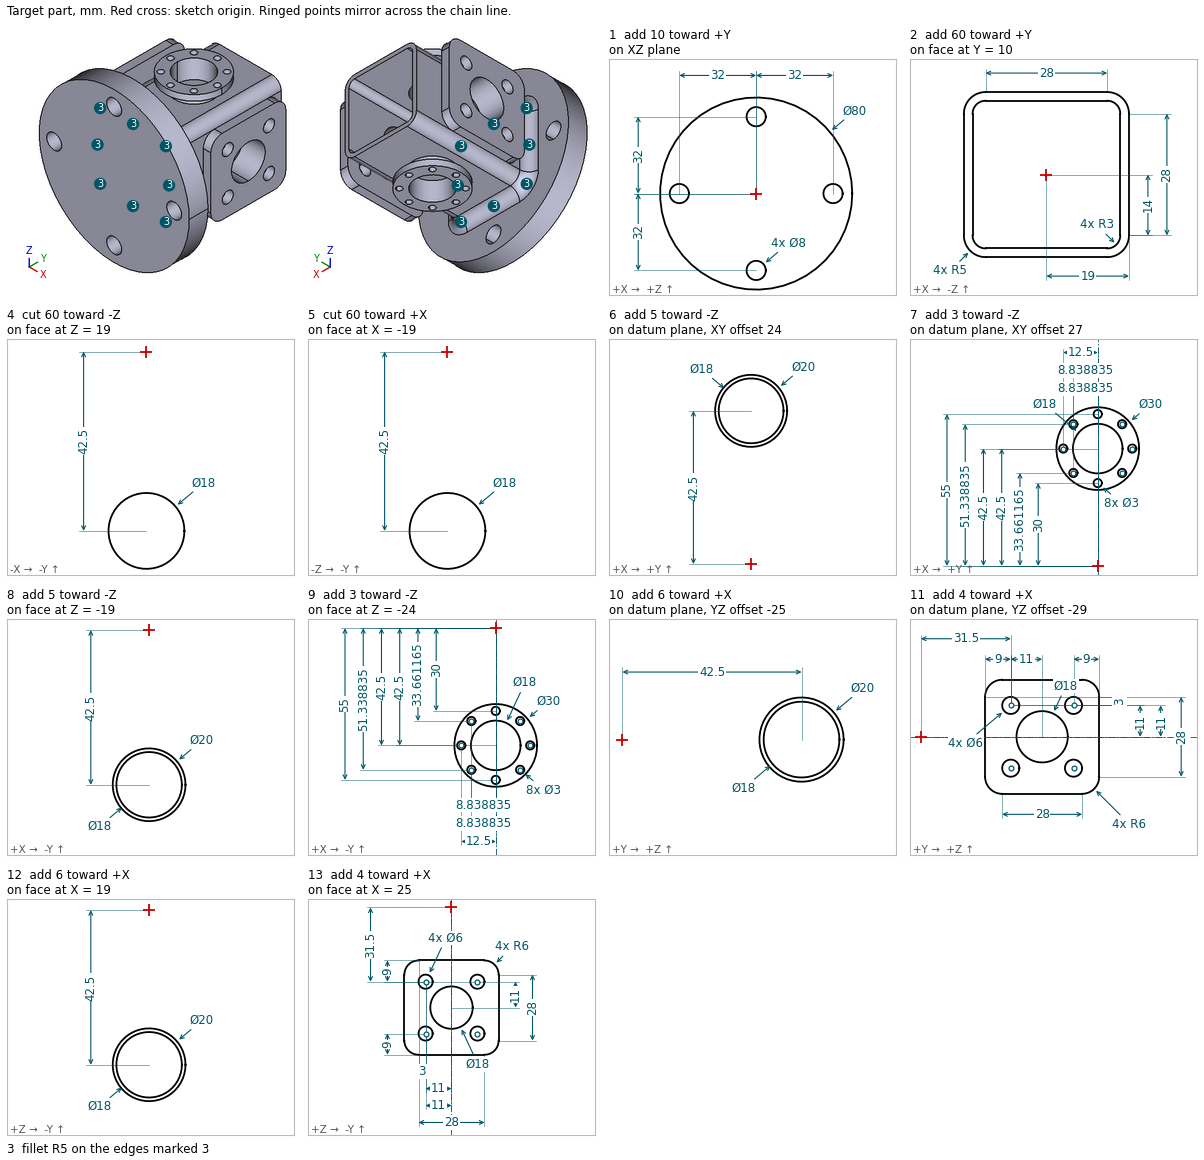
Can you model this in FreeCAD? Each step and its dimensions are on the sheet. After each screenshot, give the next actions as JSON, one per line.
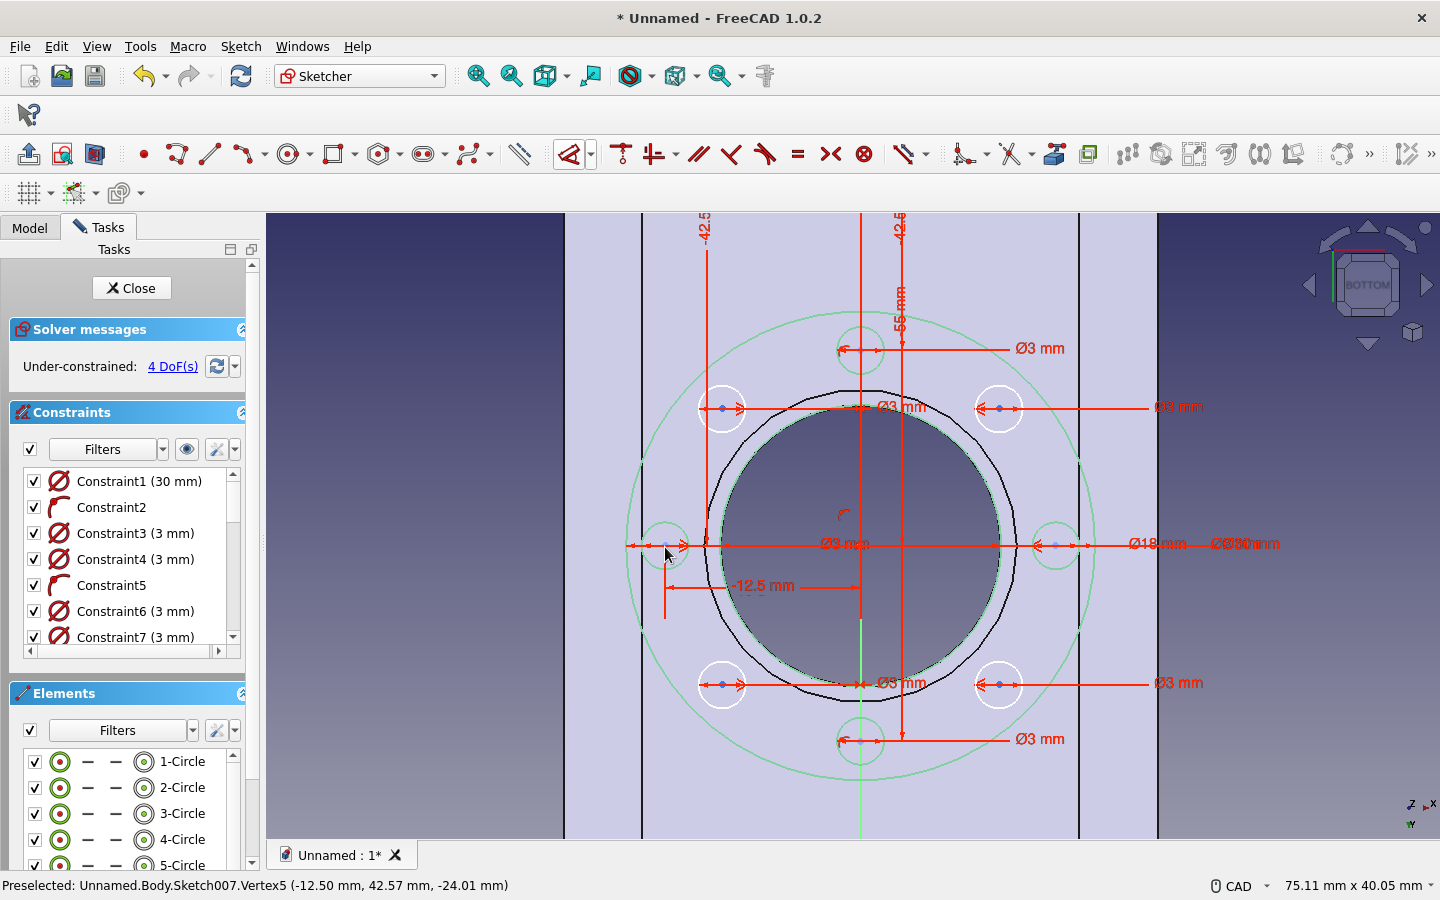
{"action": "left_click", "coordinate": [722, 685]}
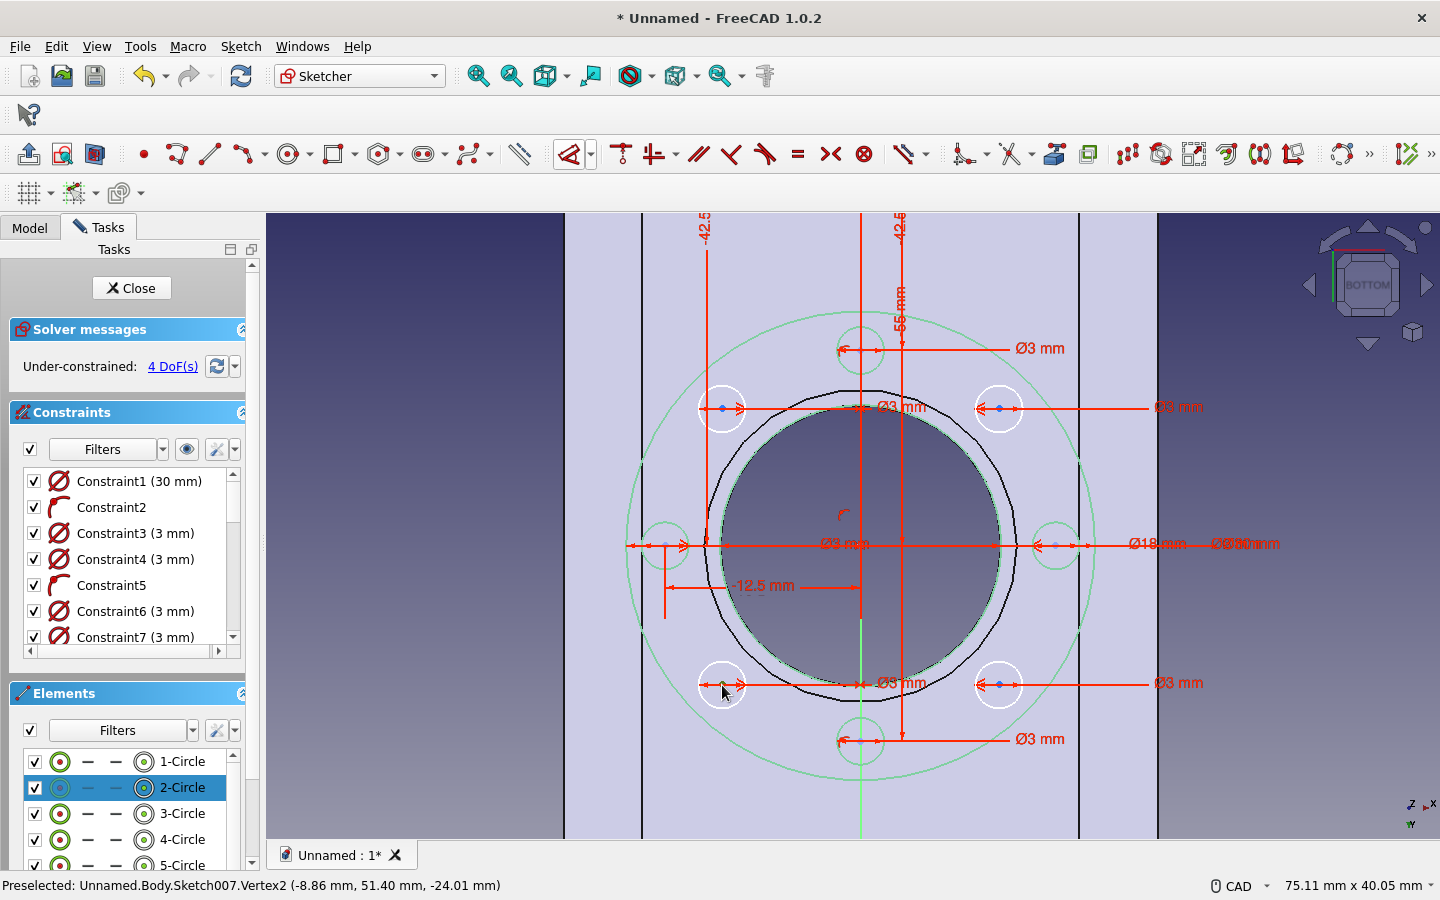
{"action": "key", "text": "l"}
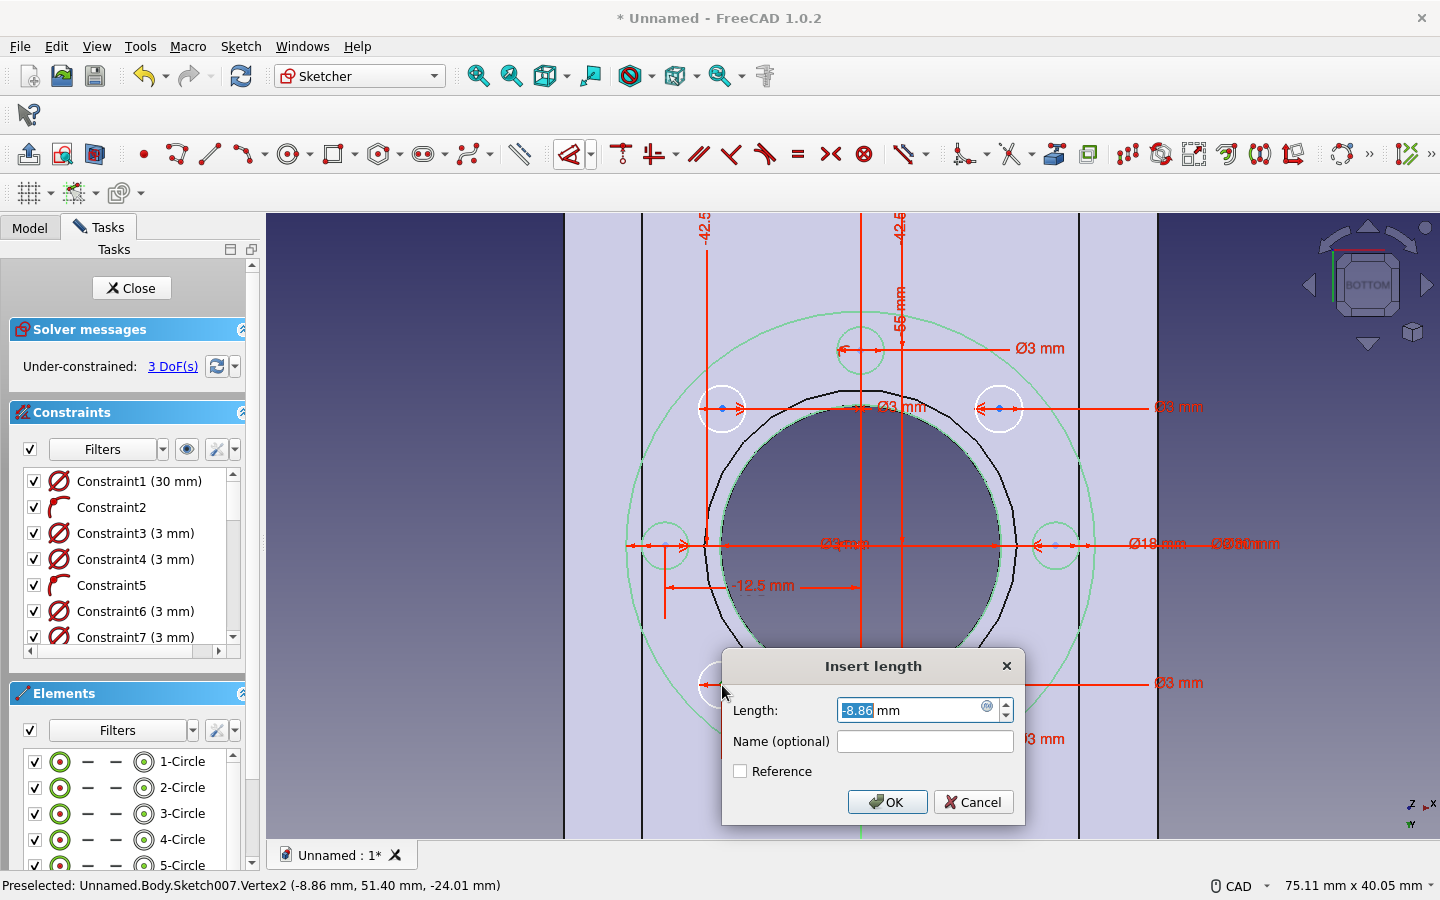
{"action": "type", "text": "-8.838835"}
{"action": "key", "text": "Return"}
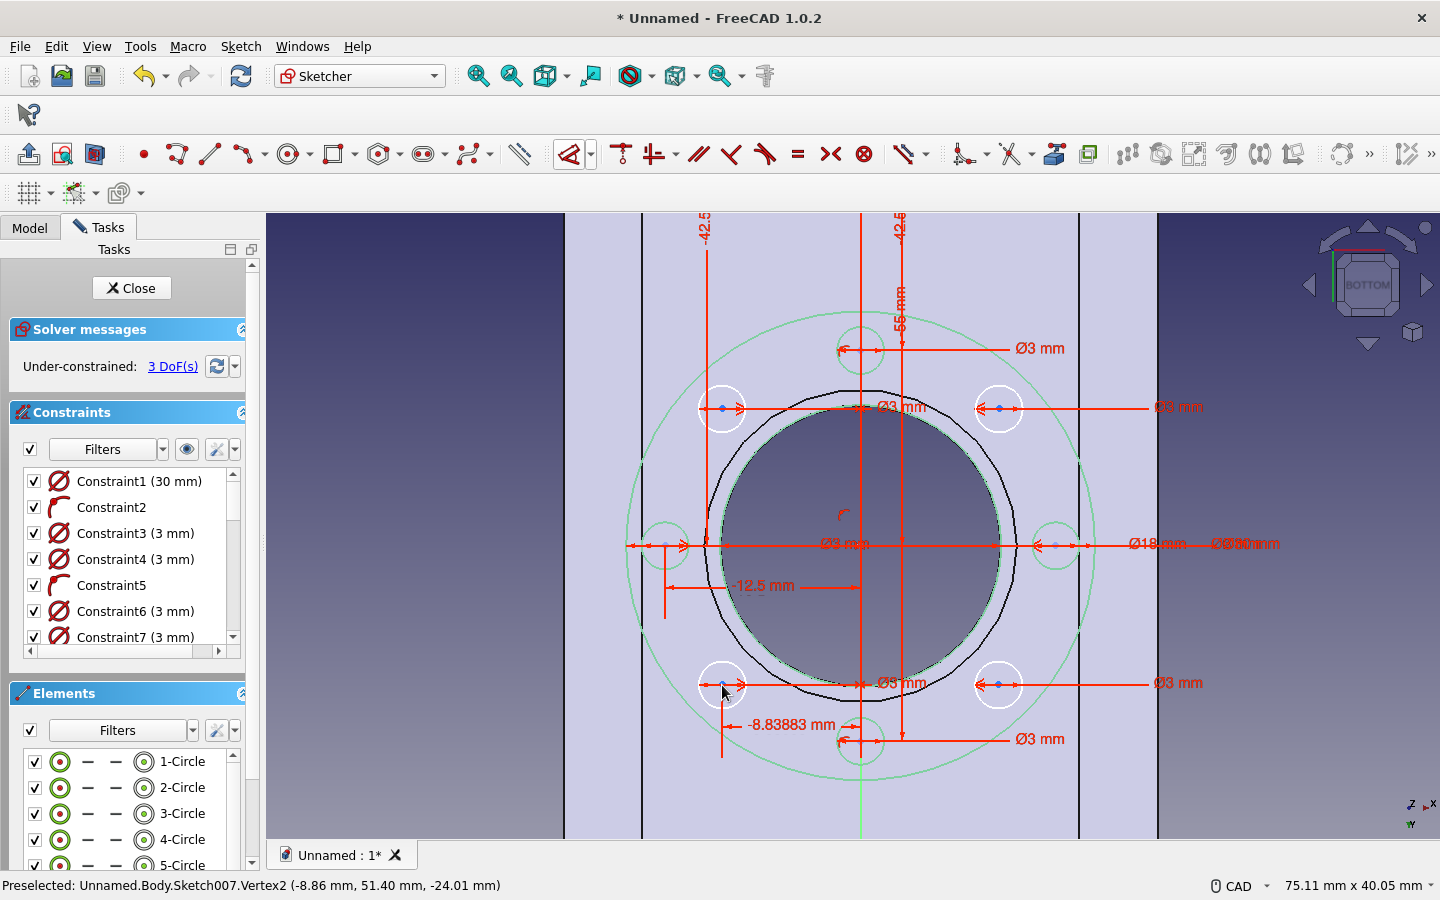
{"action": "left_click", "coordinate": [722, 409]}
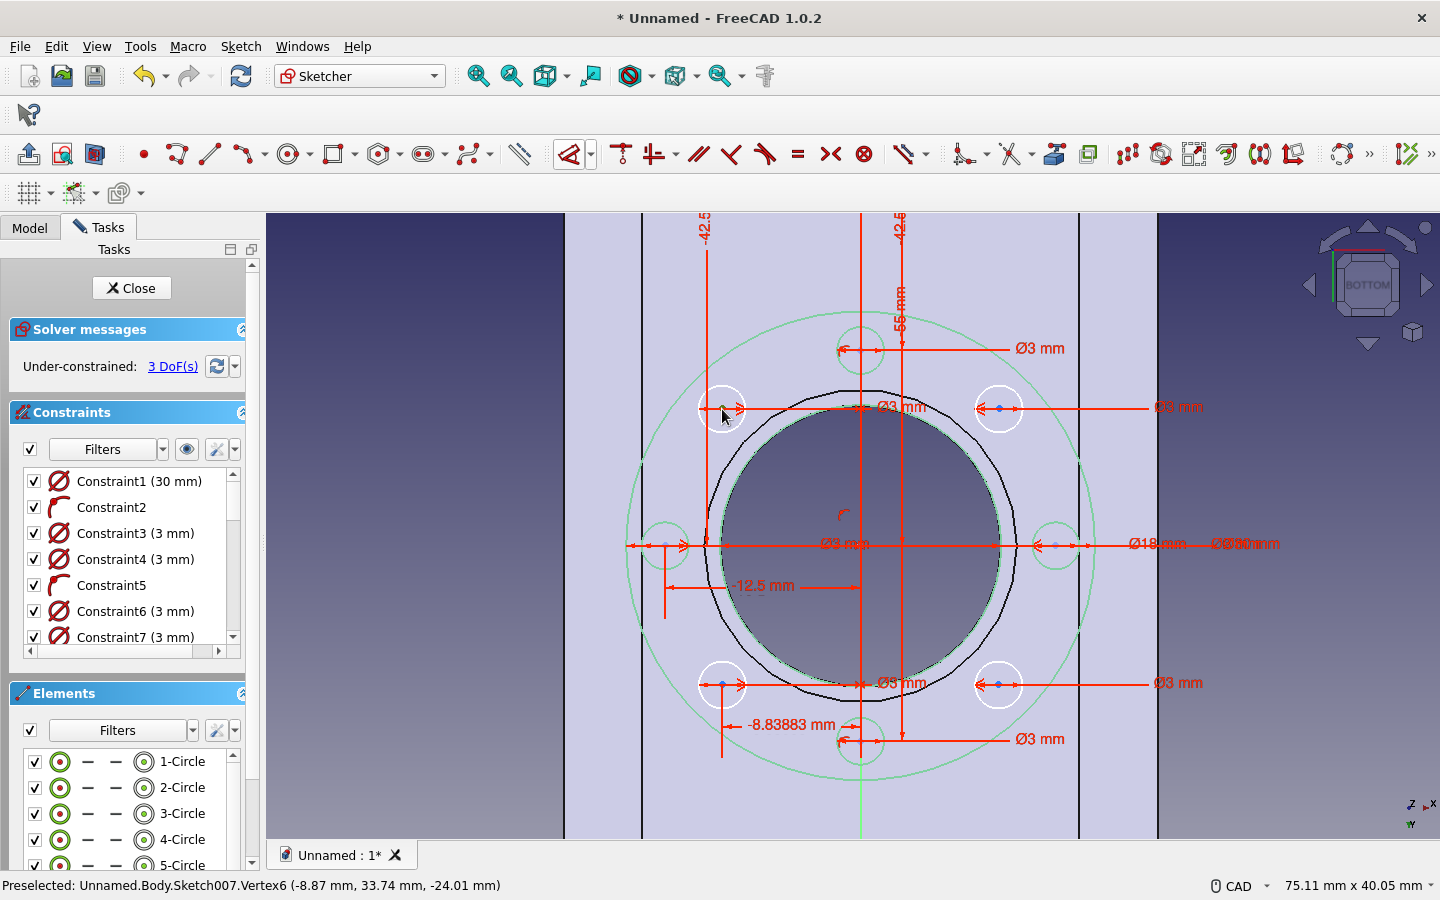
{"action": "key", "text": "l"}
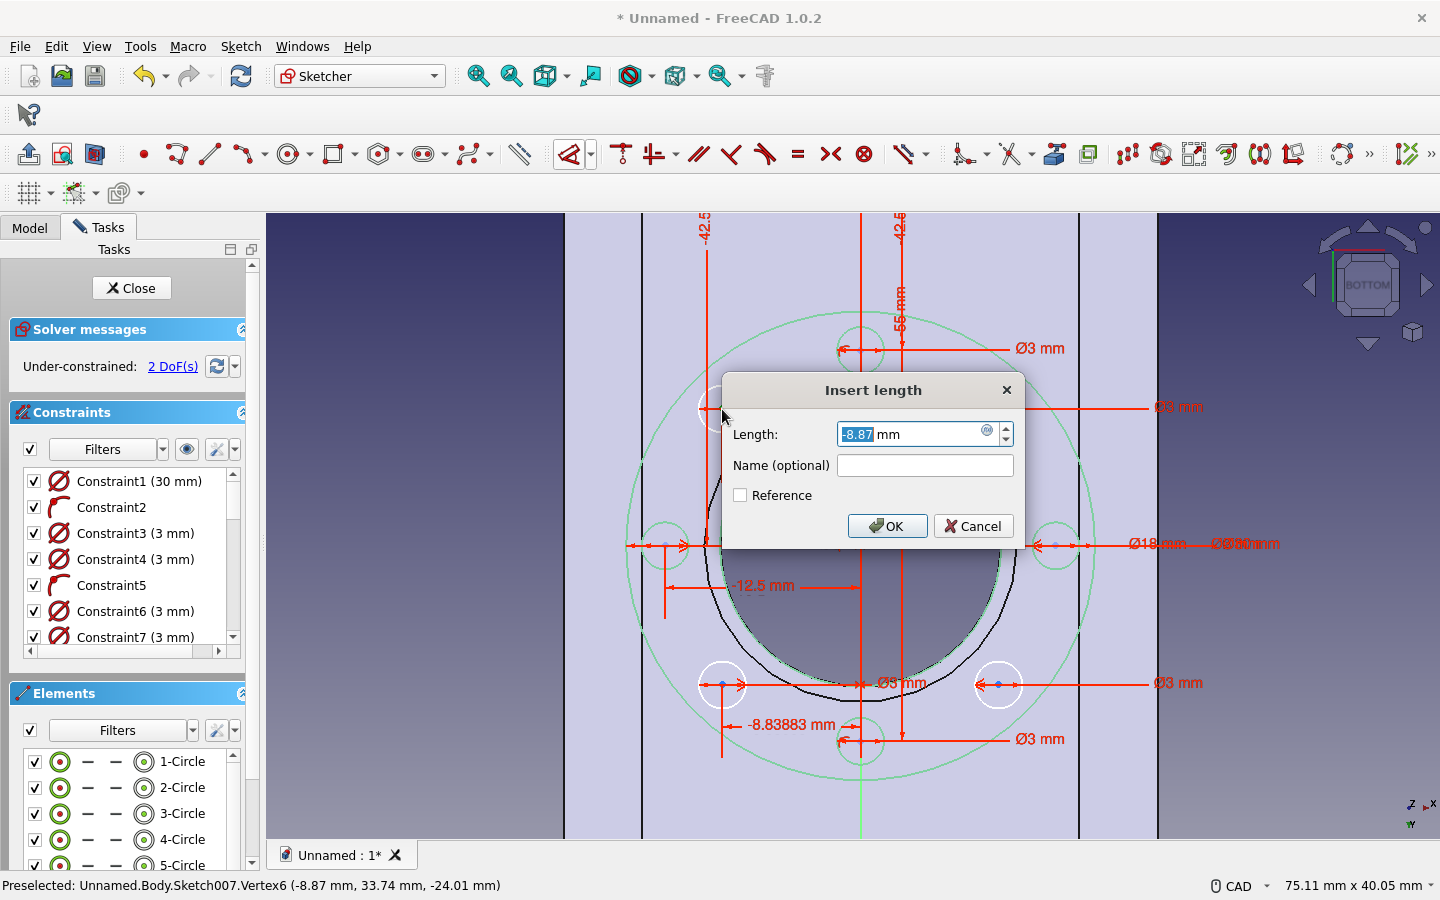
{"action": "type", "text": "-8.838835"}
{"action": "key", "text": "Return"}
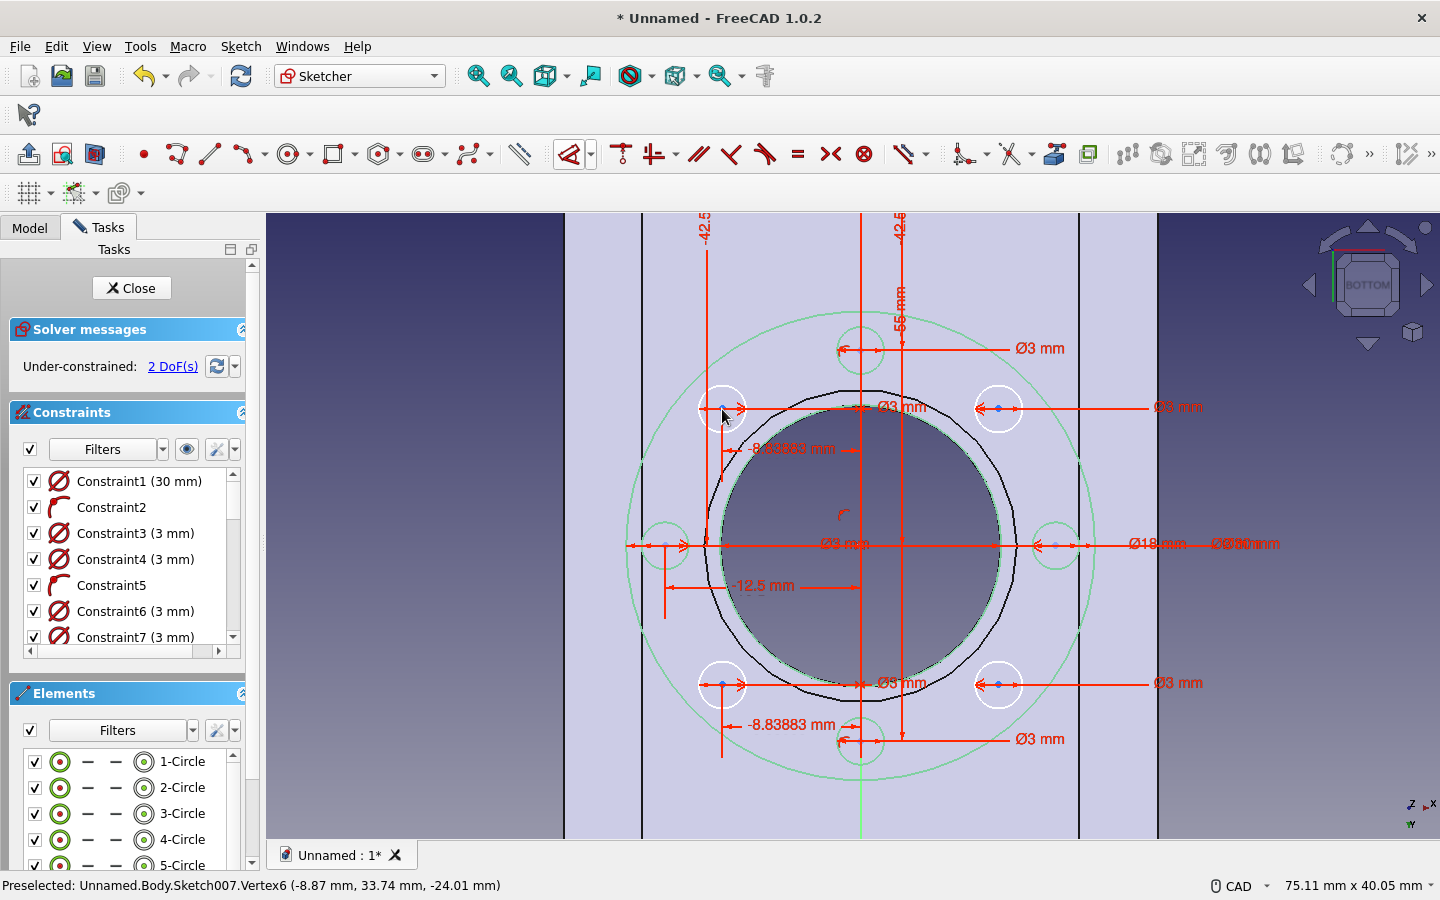
{"action": "left_click", "coordinate": [722, 685]}